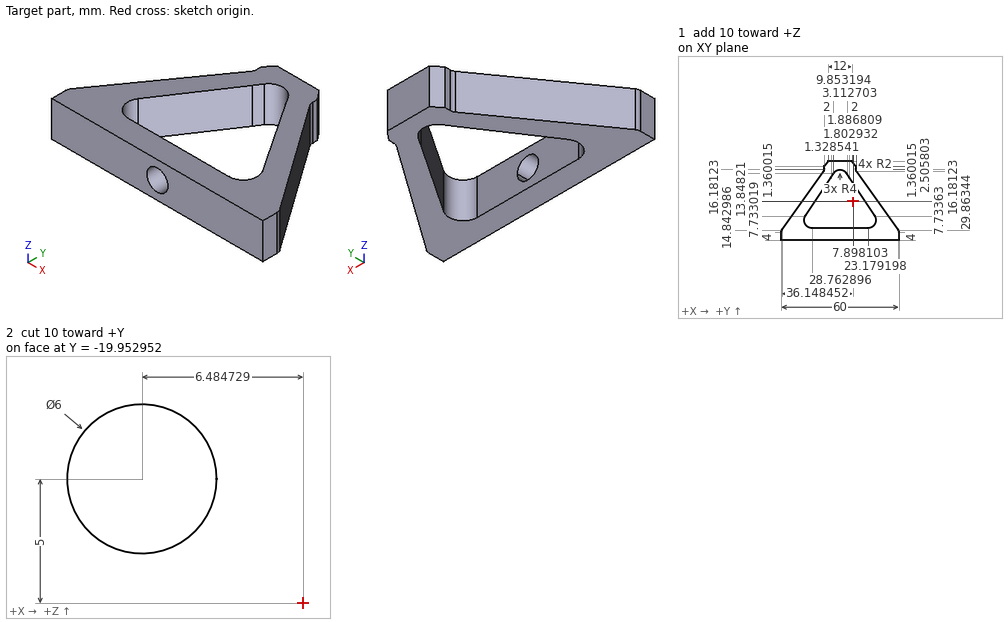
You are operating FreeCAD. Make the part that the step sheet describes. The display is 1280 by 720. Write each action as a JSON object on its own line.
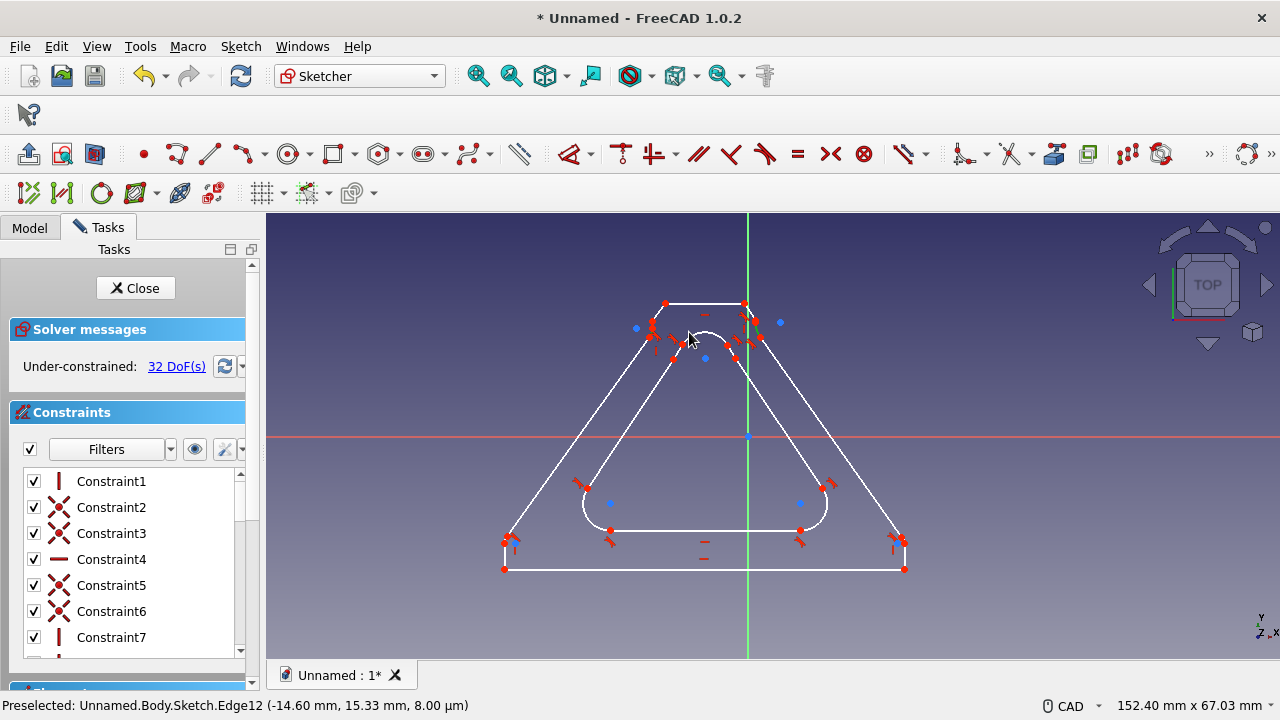
{"action": "scroll", "coordinate": [505, 539], "scroll_direction": "up", "scroll_amount": 7}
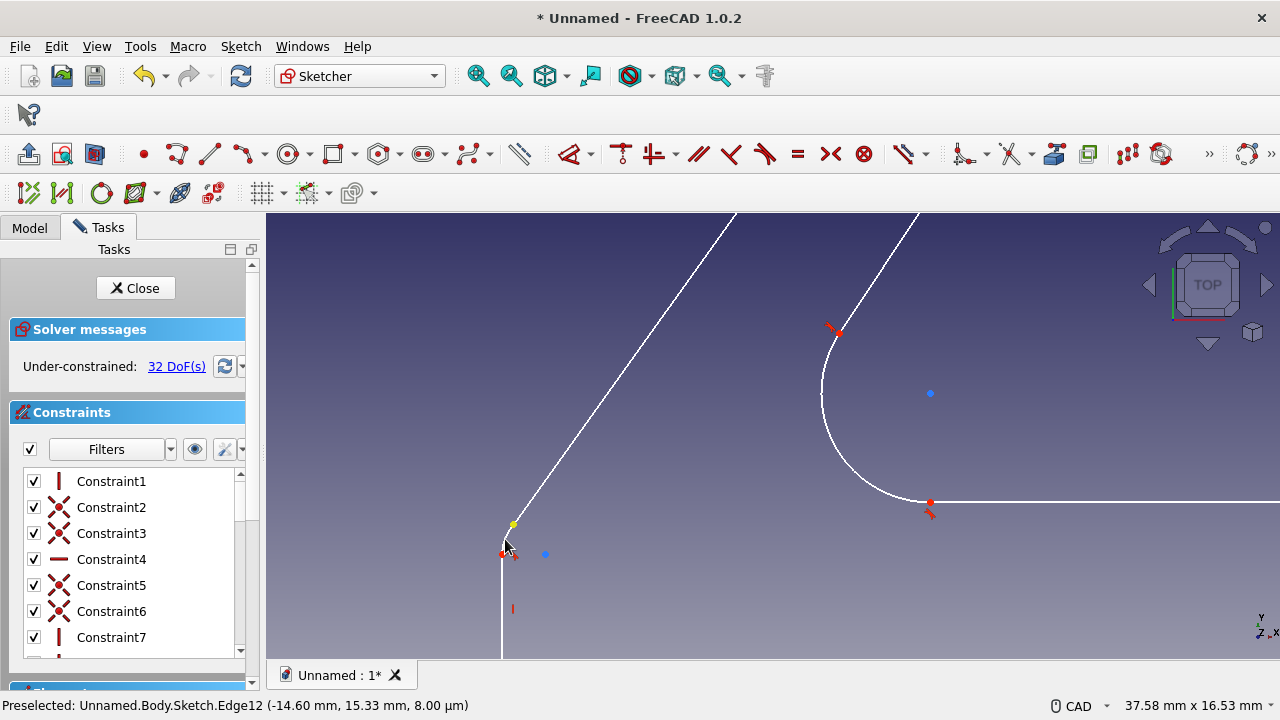
{"action": "left_click", "coordinate": [505, 538]}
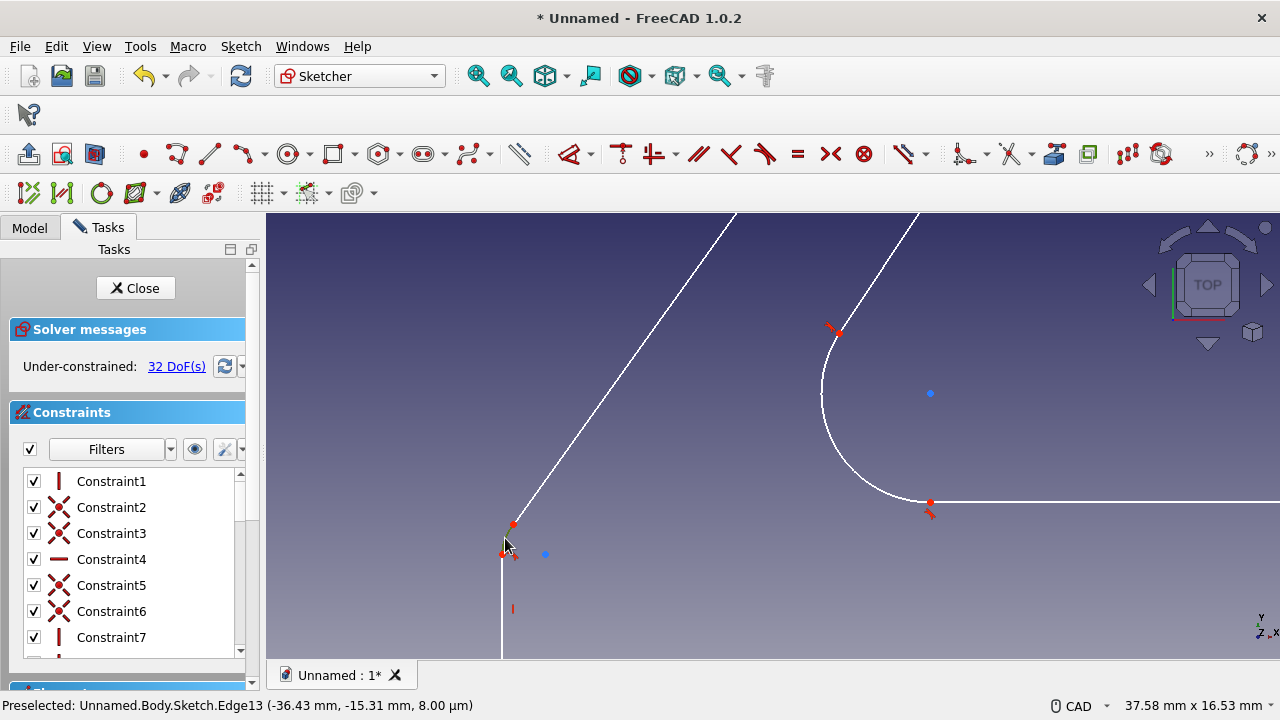
{"action": "scroll", "coordinate": [505, 539], "scroll_direction": "down", "scroll_amount": 7}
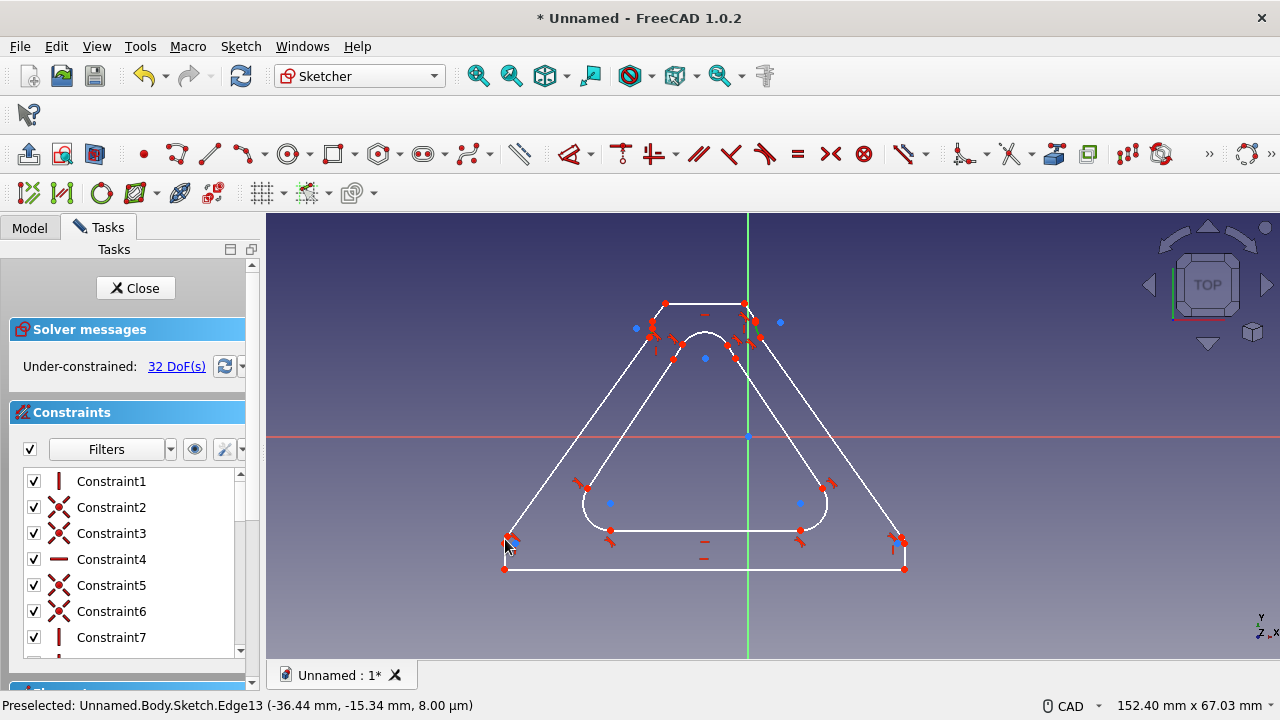
{"action": "scroll", "coordinate": [904, 540], "scroll_direction": "up", "scroll_amount": 8}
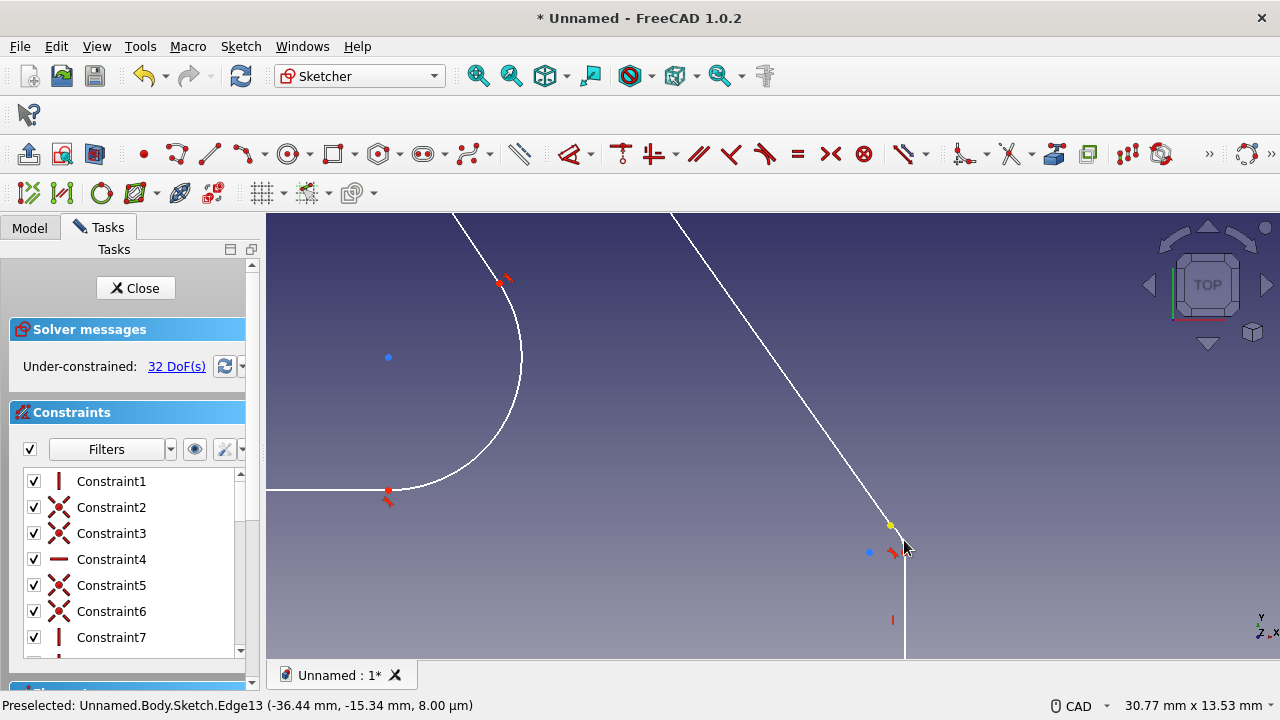
{"action": "left_click", "coordinate": [901, 537]}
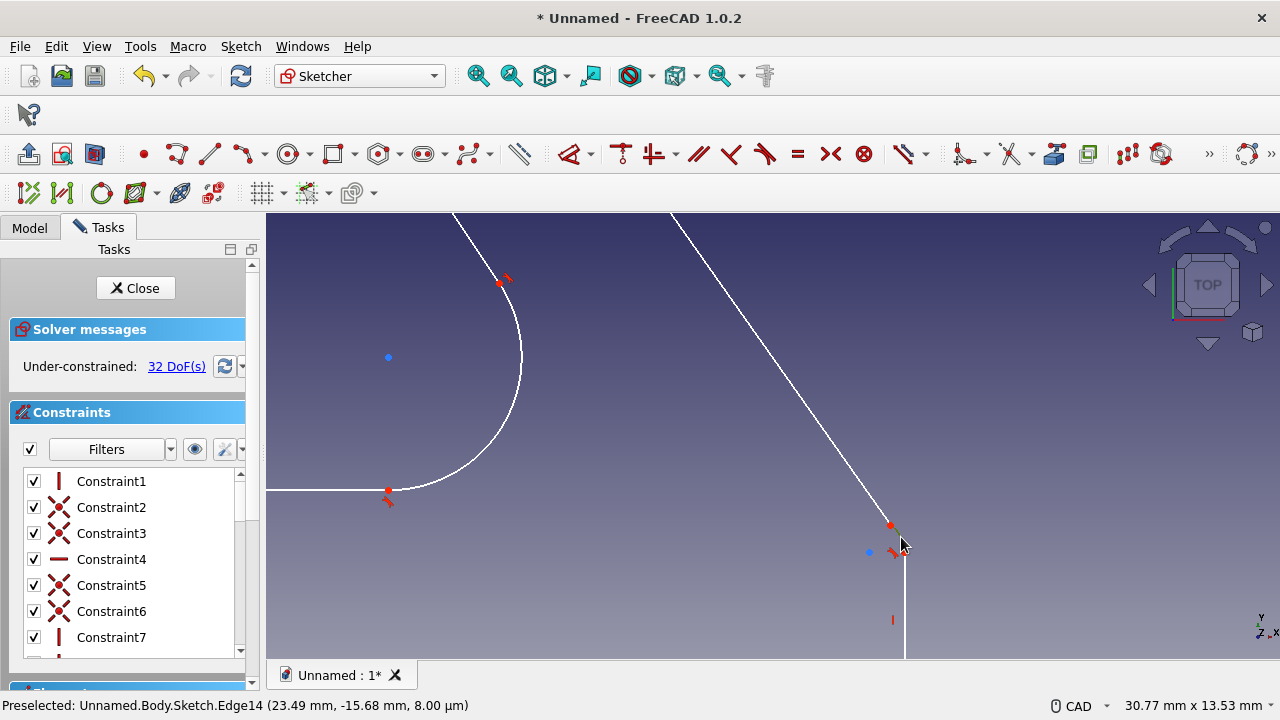
{"action": "left_click", "coordinate": [798, 154]}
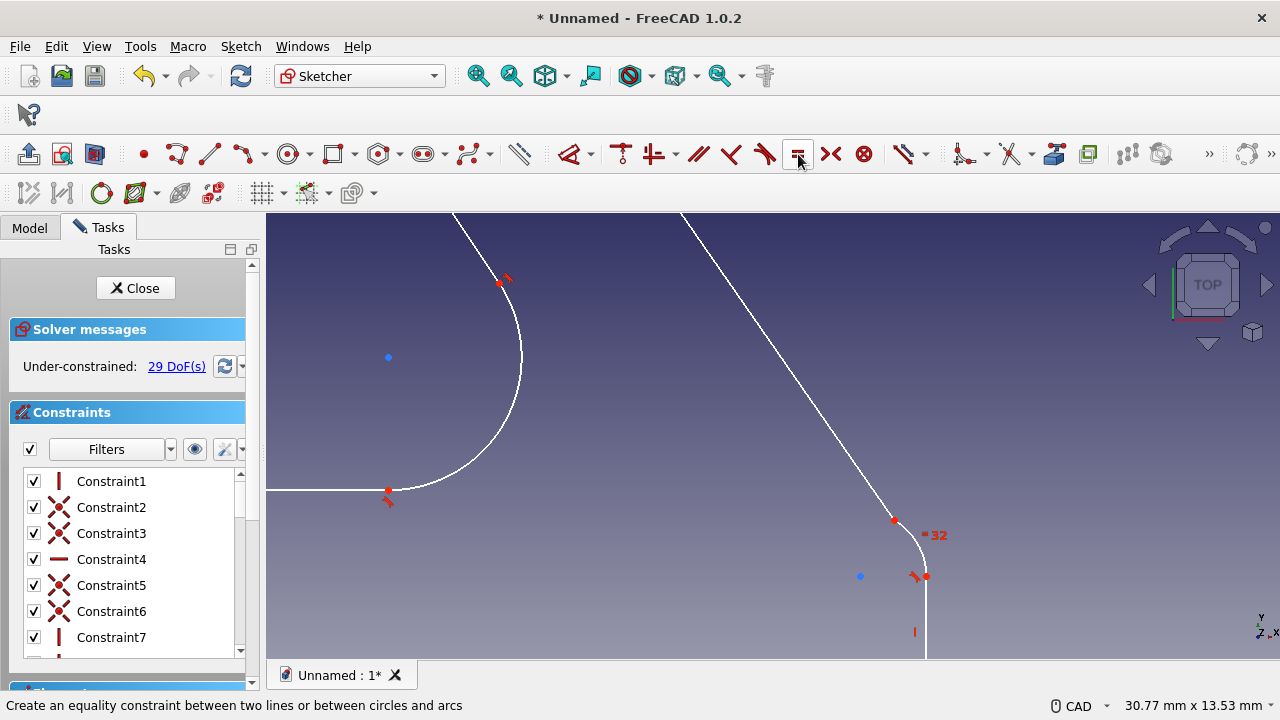
{"action": "scroll", "coordinate": [904, 540], "scroll_direction": "down", "scroll_amount": 8}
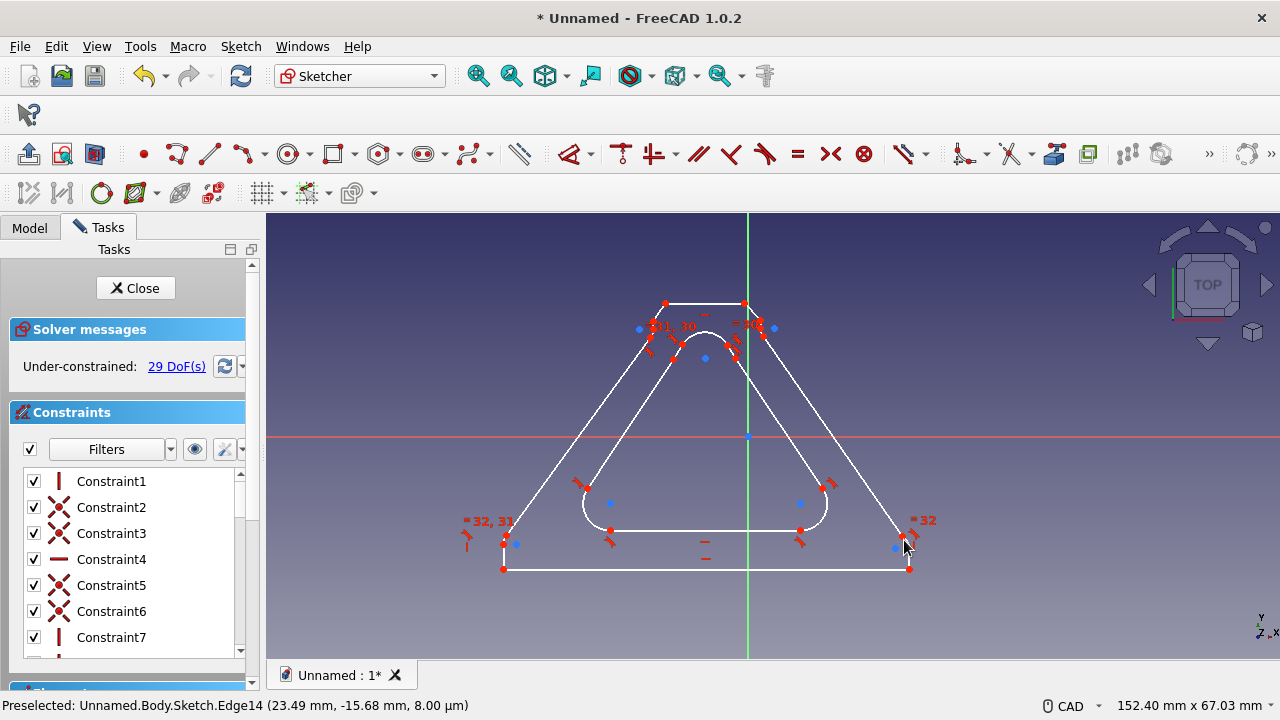
{"action": "left_click", "coordinate": [716, 335]}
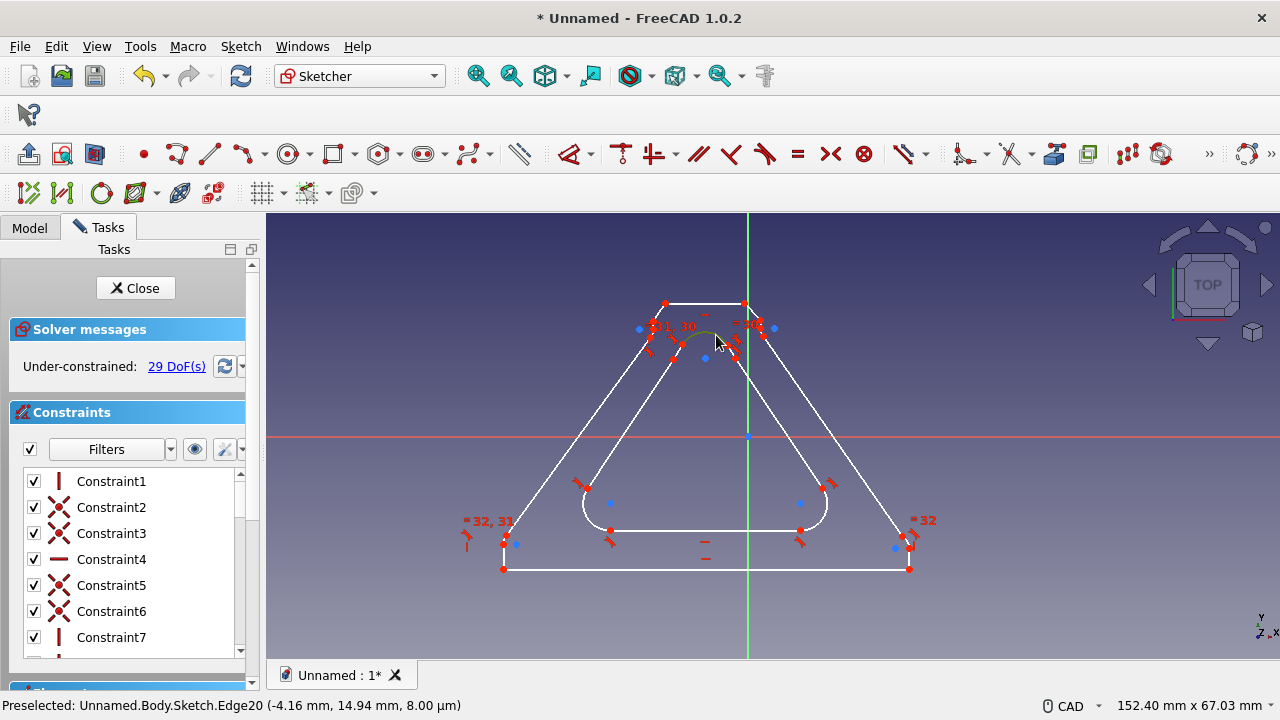
{"action": "left_click", "coordinate": [817, 525]}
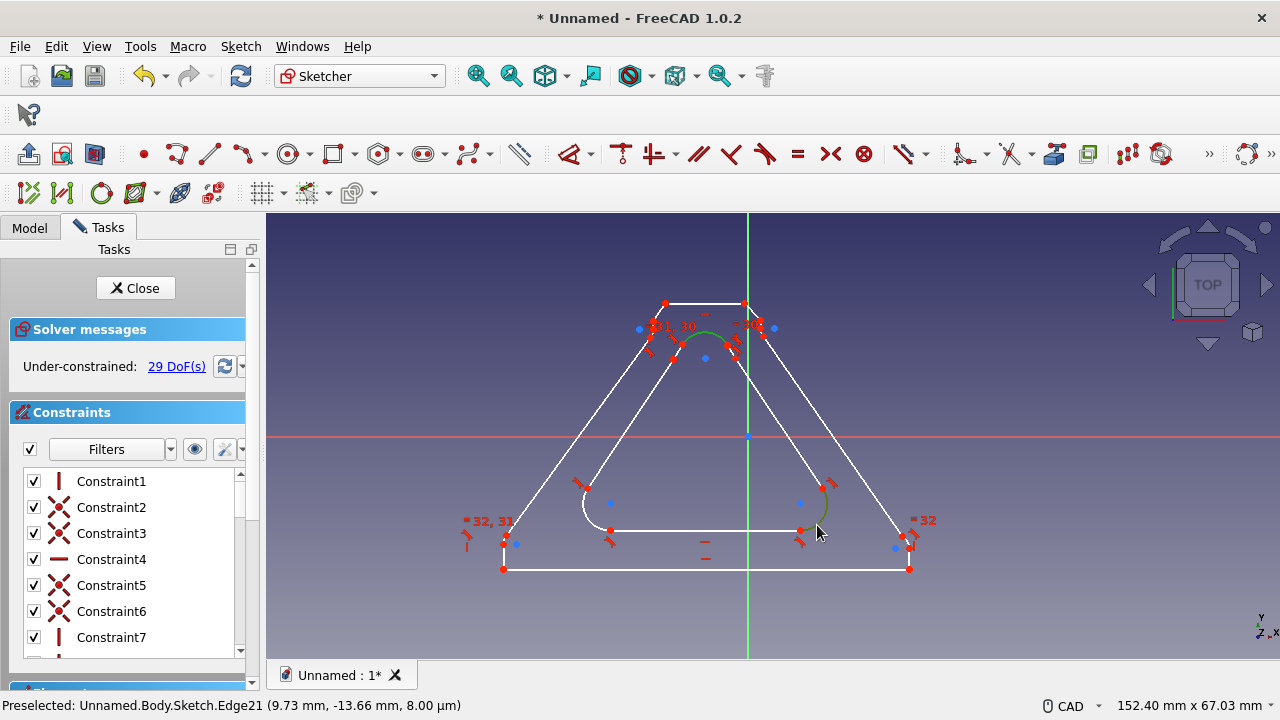
{"action": "left_click", "coordinate": [583, 505]}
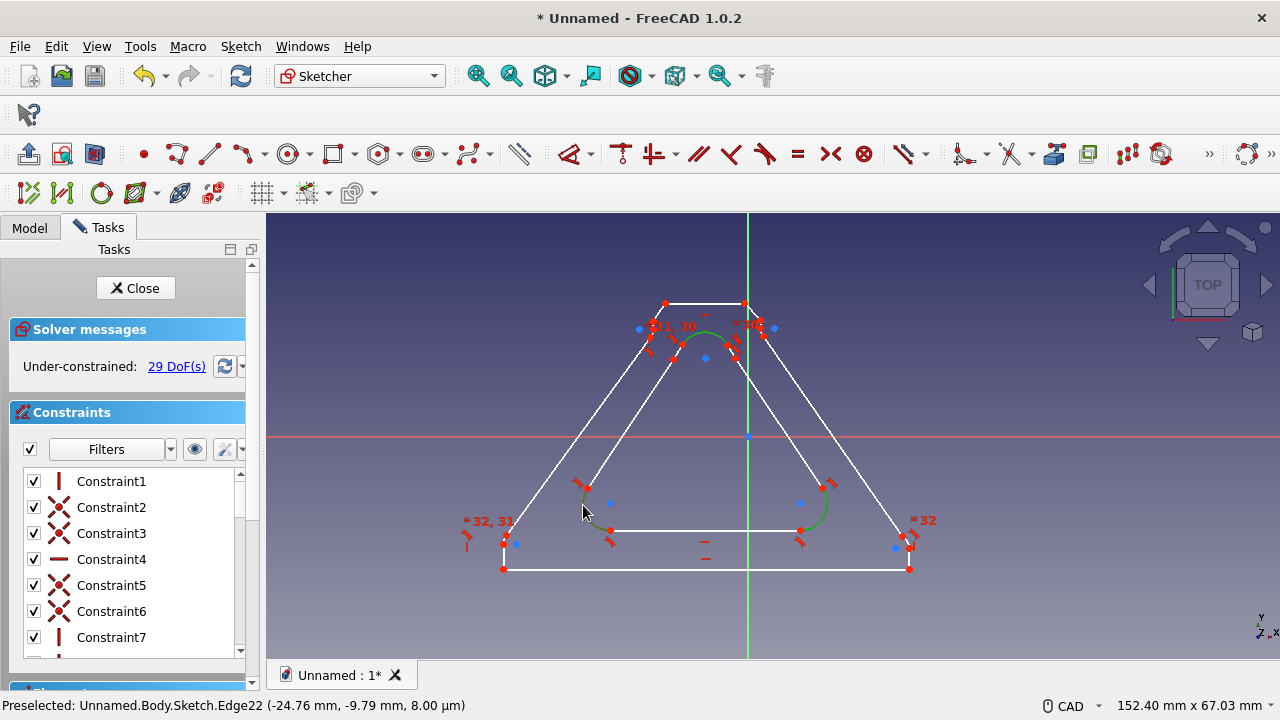
{"action": "left_click", "coordinate": [798, 154]}